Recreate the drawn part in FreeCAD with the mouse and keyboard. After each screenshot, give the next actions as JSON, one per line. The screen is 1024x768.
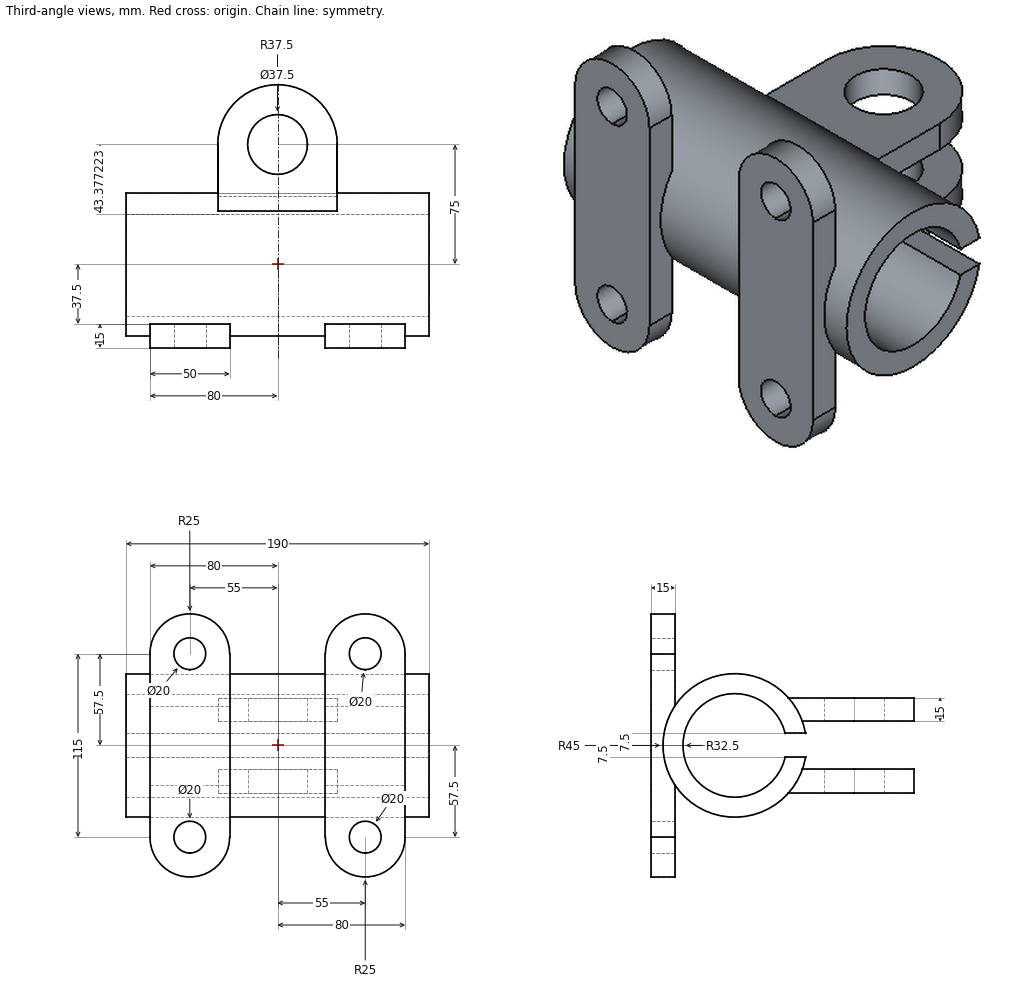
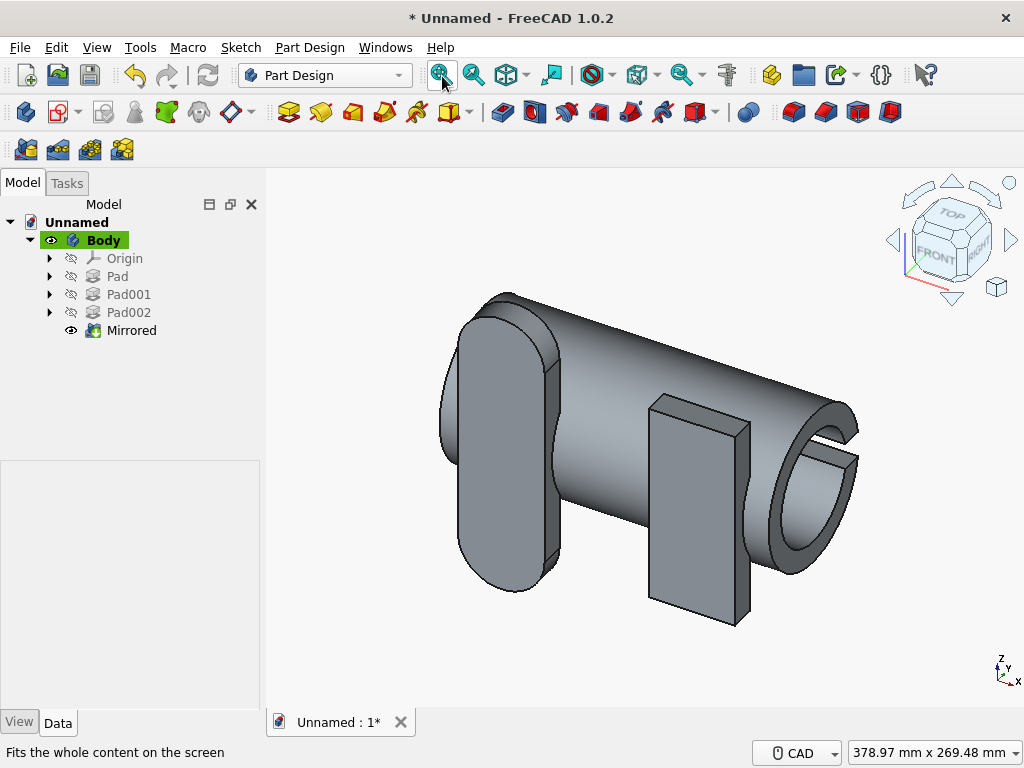
{"action": "left_click", "coordinate": [116, 312]}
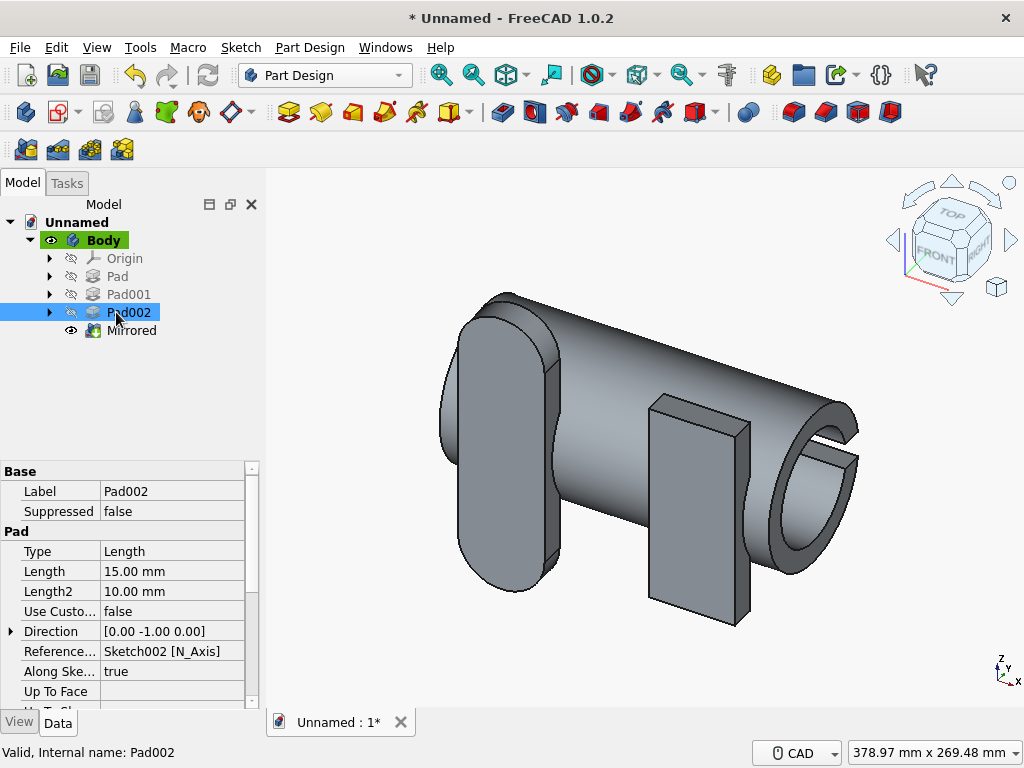
{"action": "left_click", "coordinate": [26, 150]}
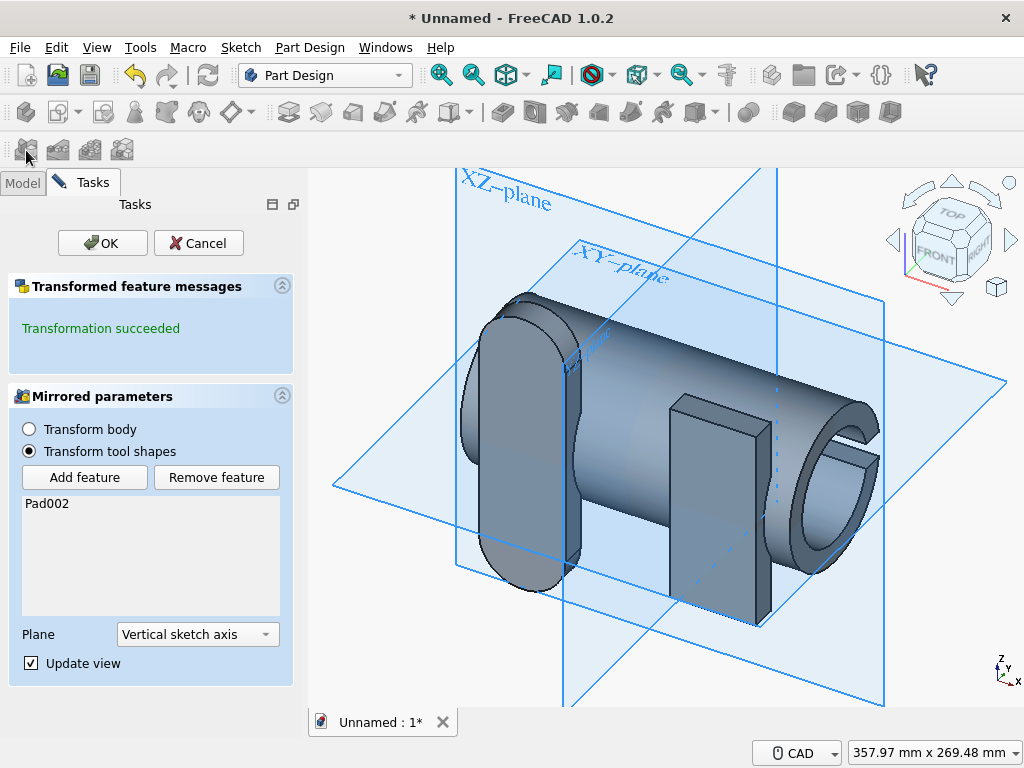
{"action": "left_click", "coordinate": [198, 634]}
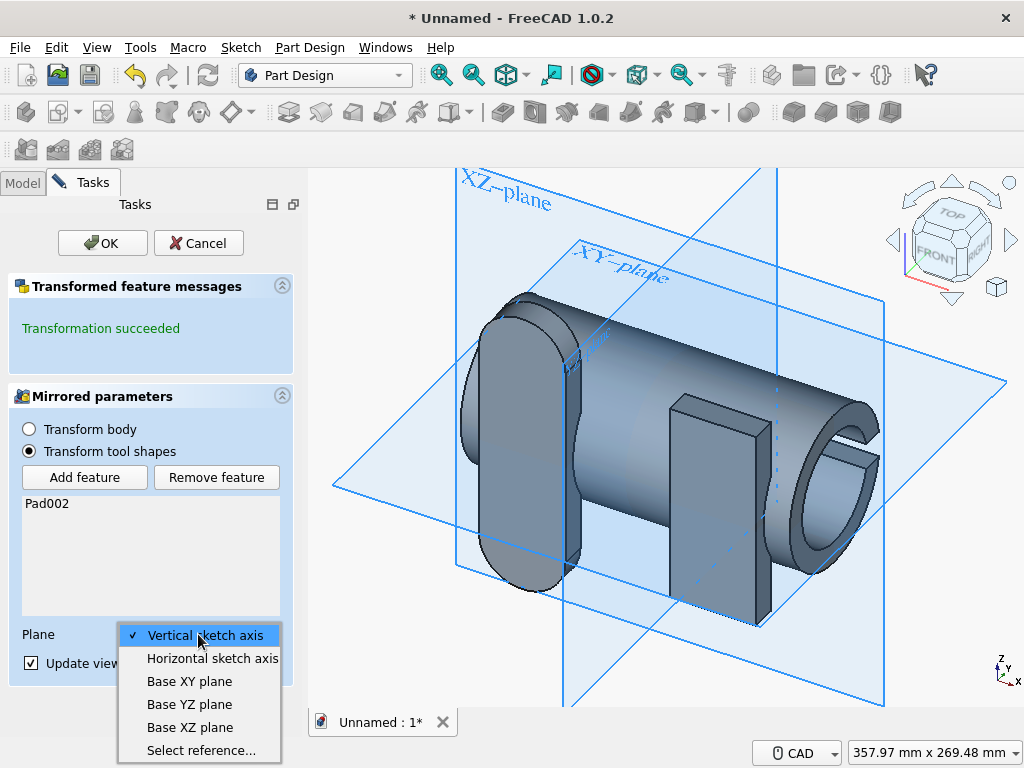
{"action": "left_click", "coordinate": [198, 704]}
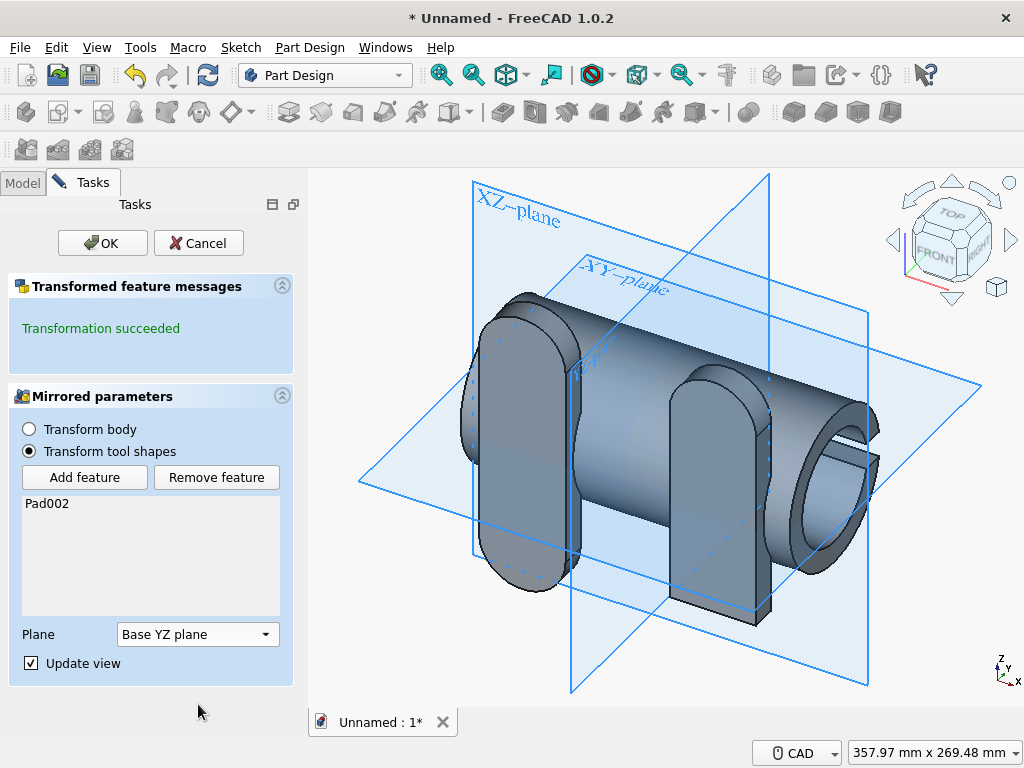
{"action": "left_click", "coordinate": [103, 243]}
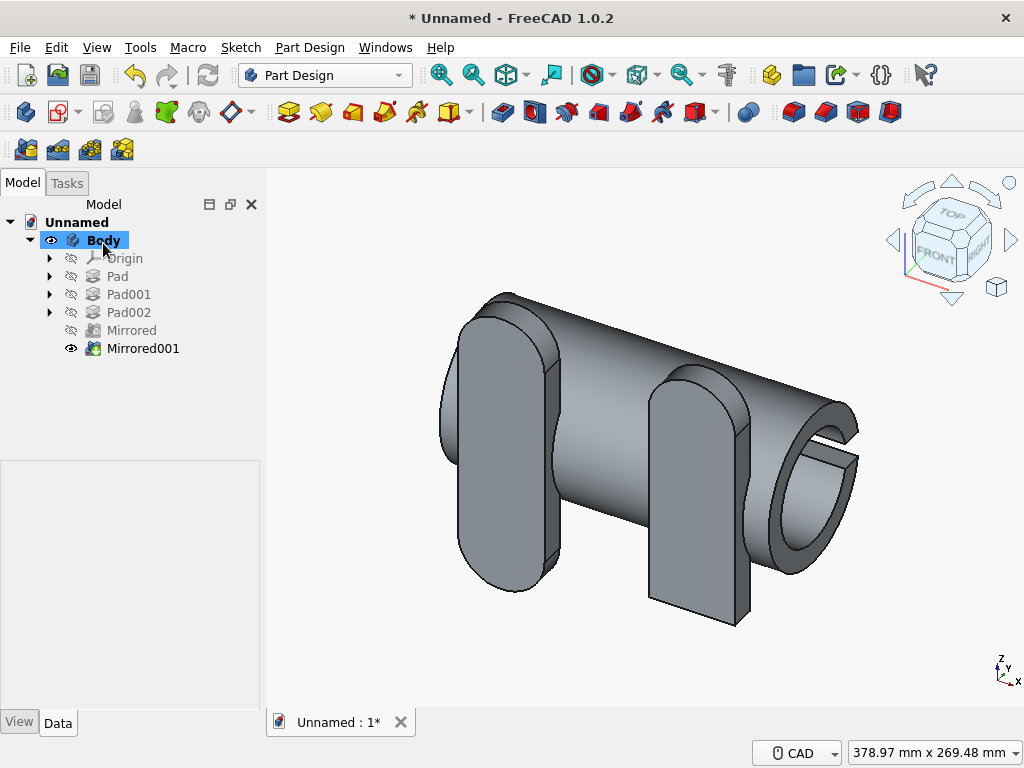
{"action": "left_click", "coordinate": [501, 453]}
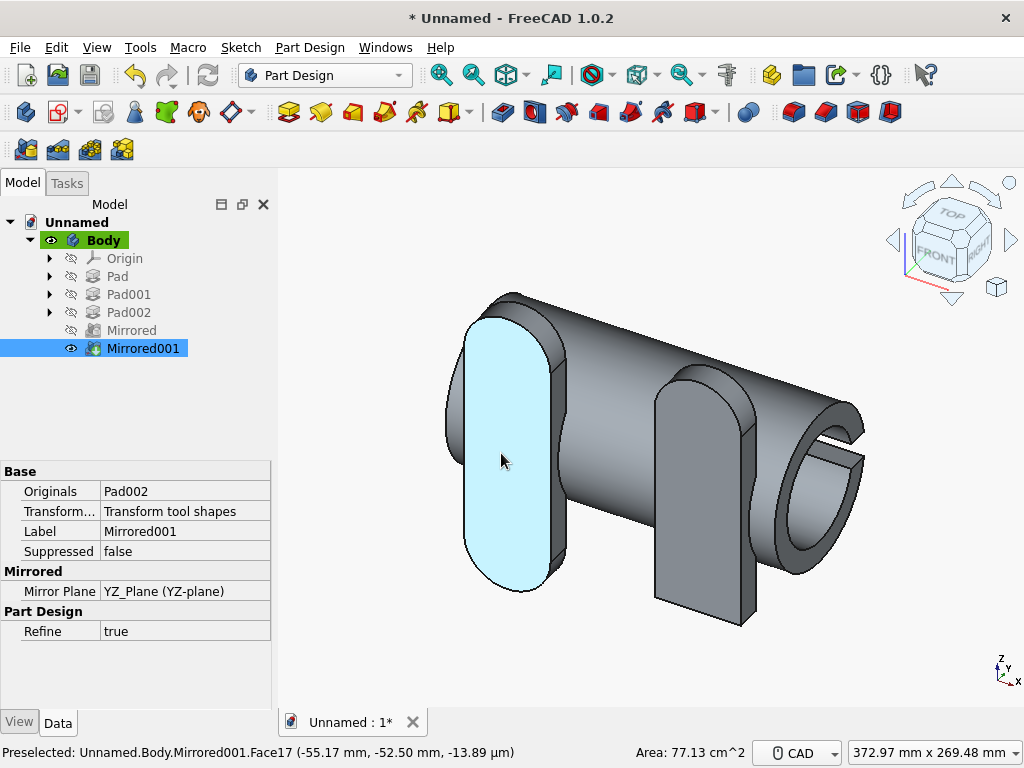
{"action": "left_click", "coordinate": [58, 112]}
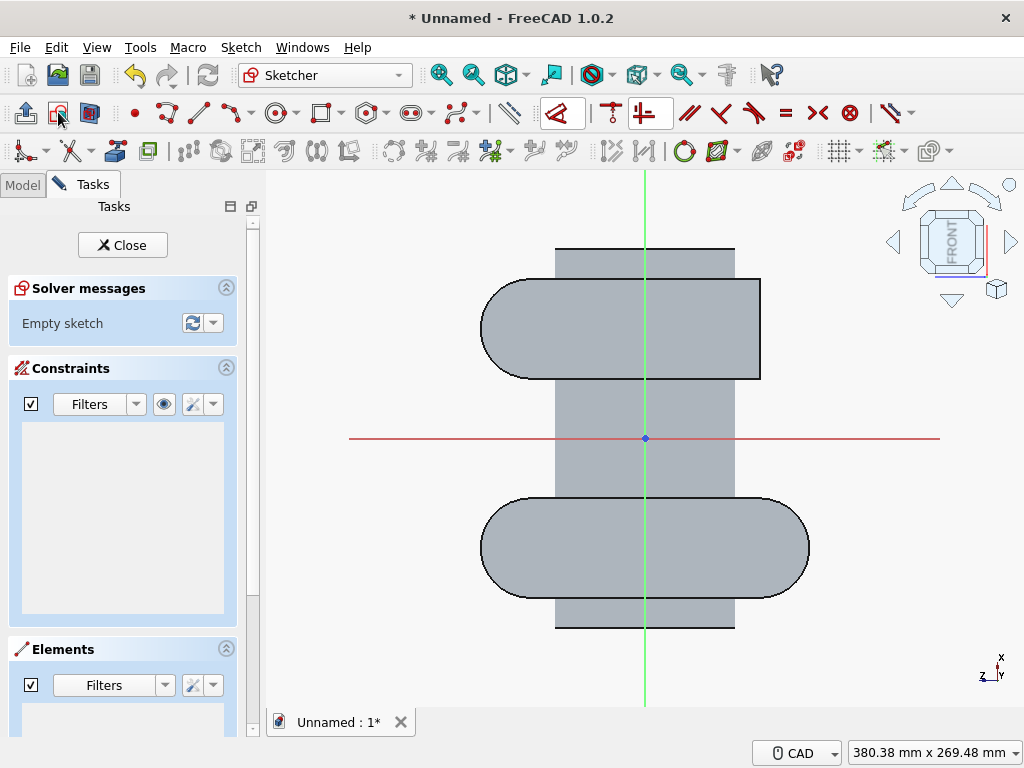
{"action": "scroll", "coordinate": [850, 294], "scroll_direction": "up", "scroll_amount": 4}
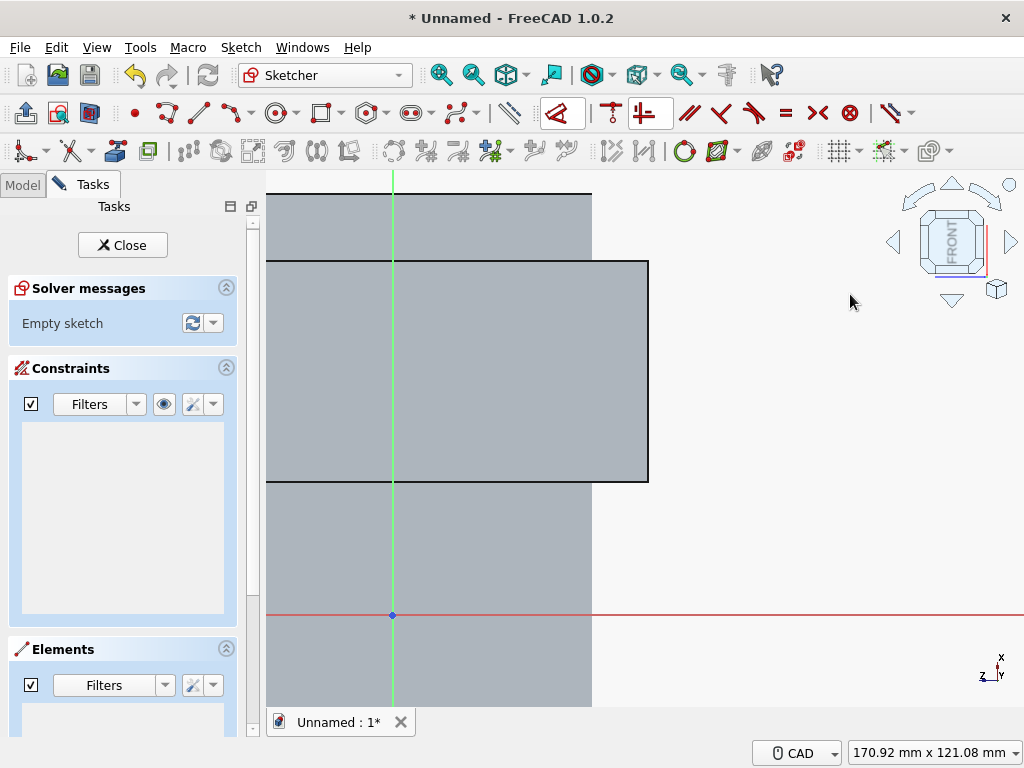
{"action": "left_click", "coordinate": [200, 114]}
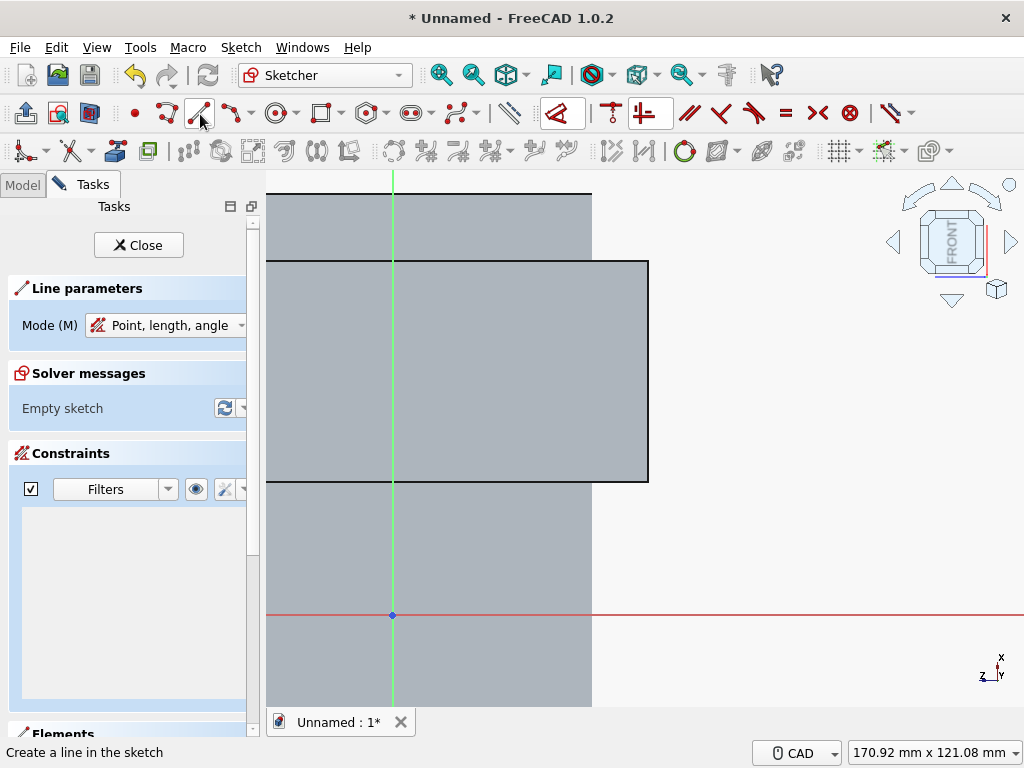
{"action": "left_click", "coordinate": [648, 261]}
{"action": "left_click", "coordinate": [648, 482]}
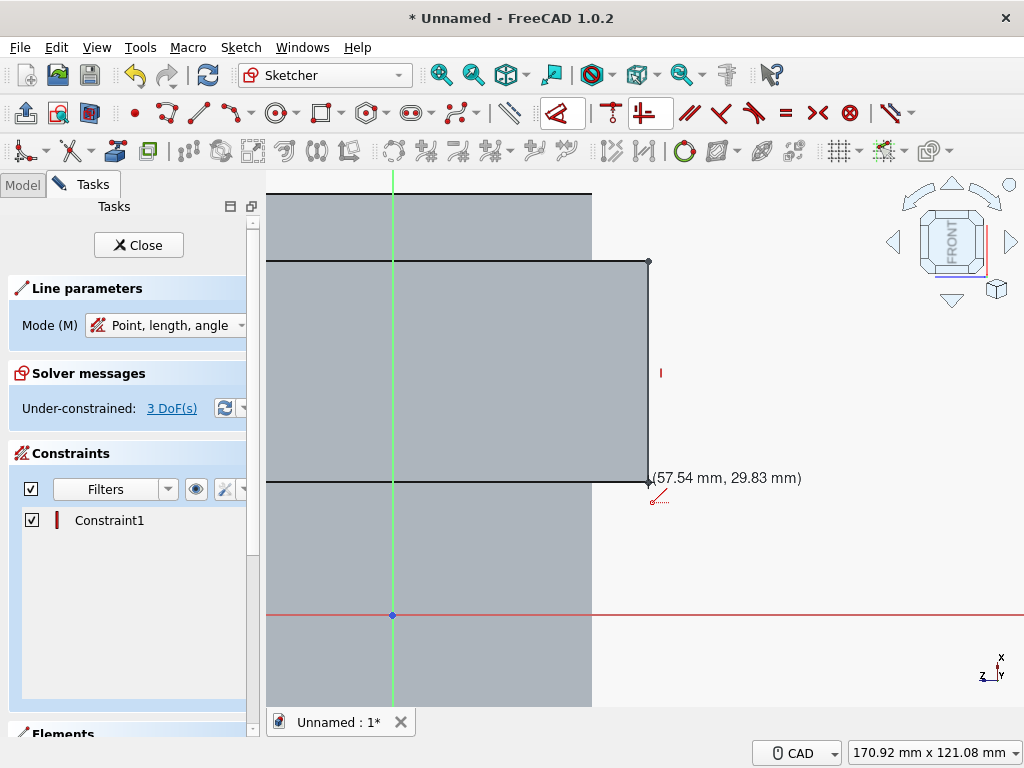
{"action": "left_click", "coordinate": [232, 114]}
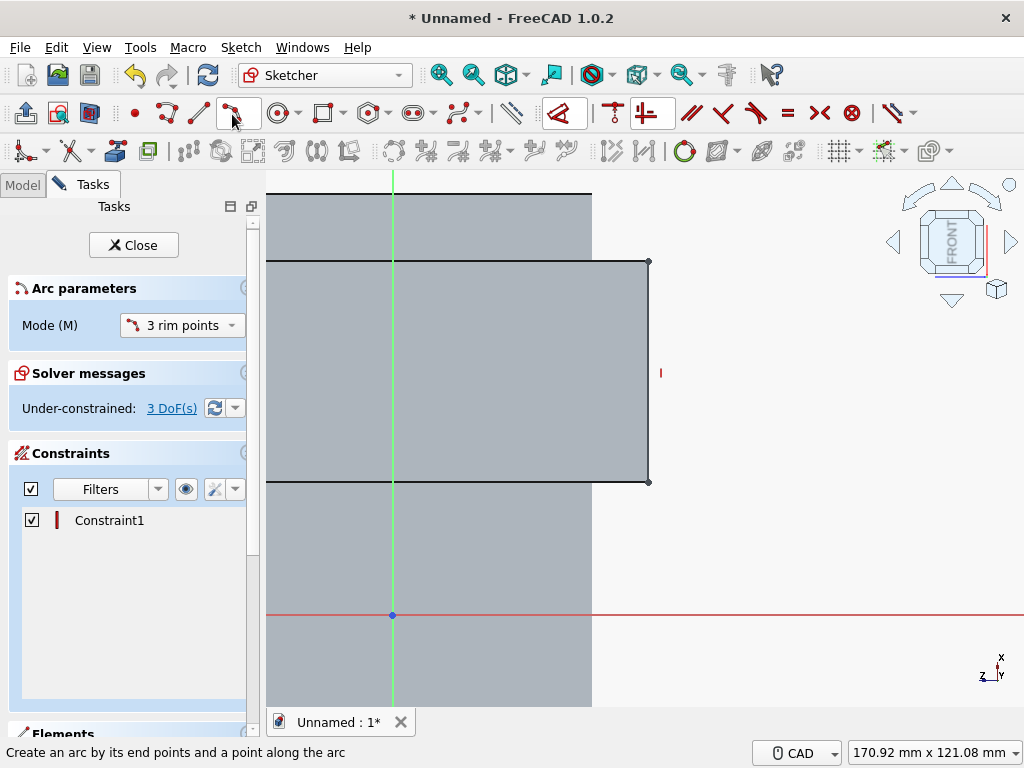
{"action": "left_click", "coordinate": [648, 483]}
{"action": "left_click", "coordinate": [648, 262]}
{"action": "left_click", "coordinate": [759, 371]}
{"action": "key", "text": "Escape"}